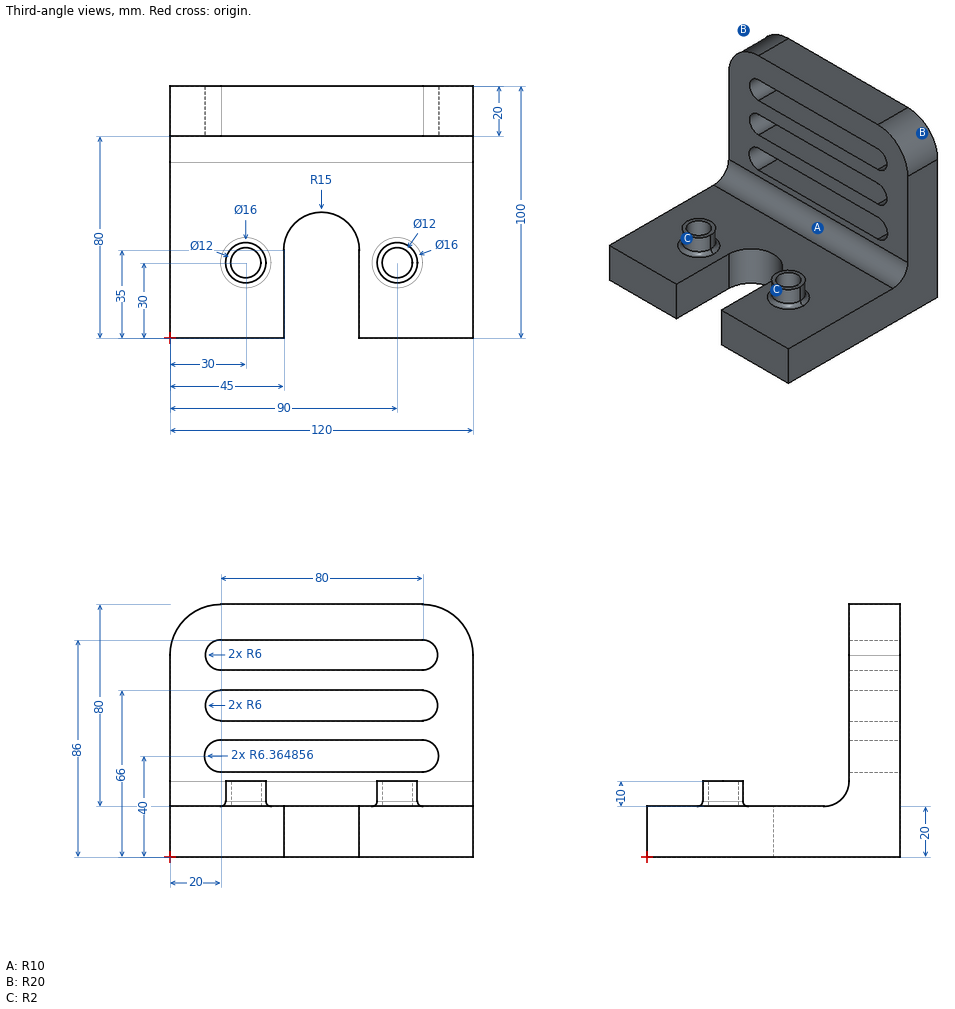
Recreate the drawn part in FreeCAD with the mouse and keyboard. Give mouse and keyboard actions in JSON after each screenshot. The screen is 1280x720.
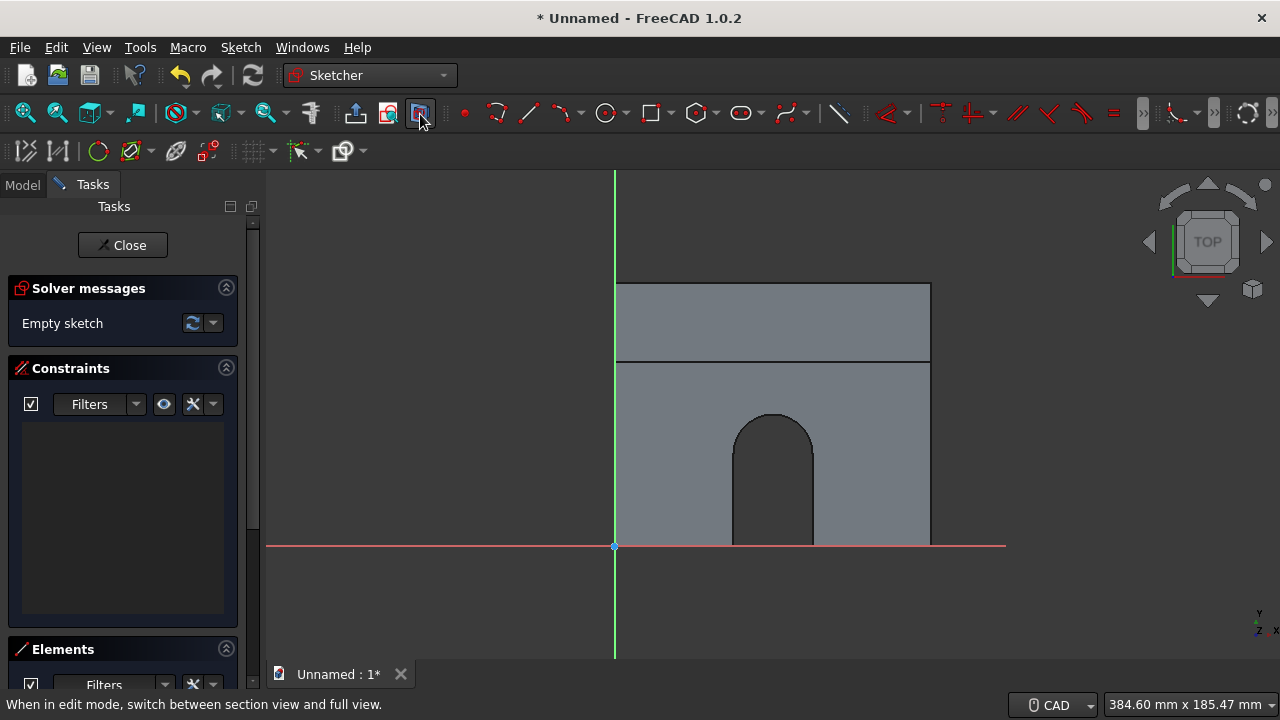
{"action": "scroll", "coordinate": [648, 531], "scroll_direction": "up", "scroll_amount": 6}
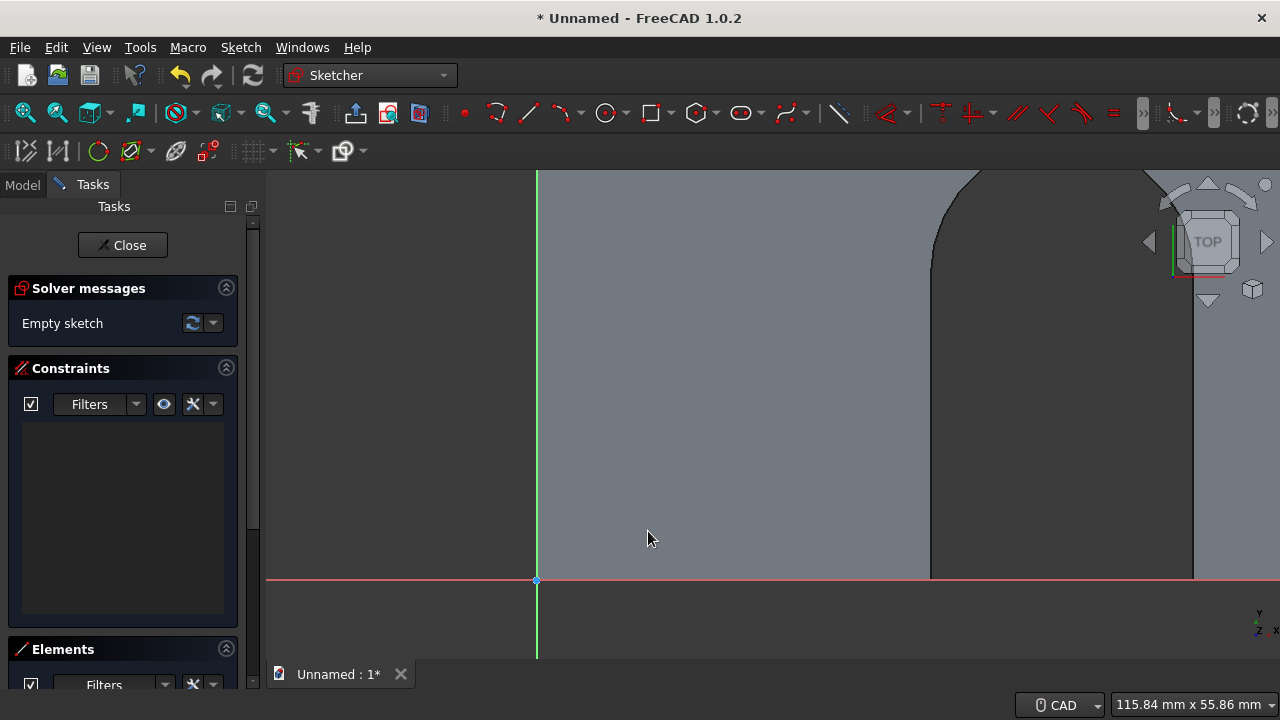
{"action": "left_click", "coordinate": [606, 114]}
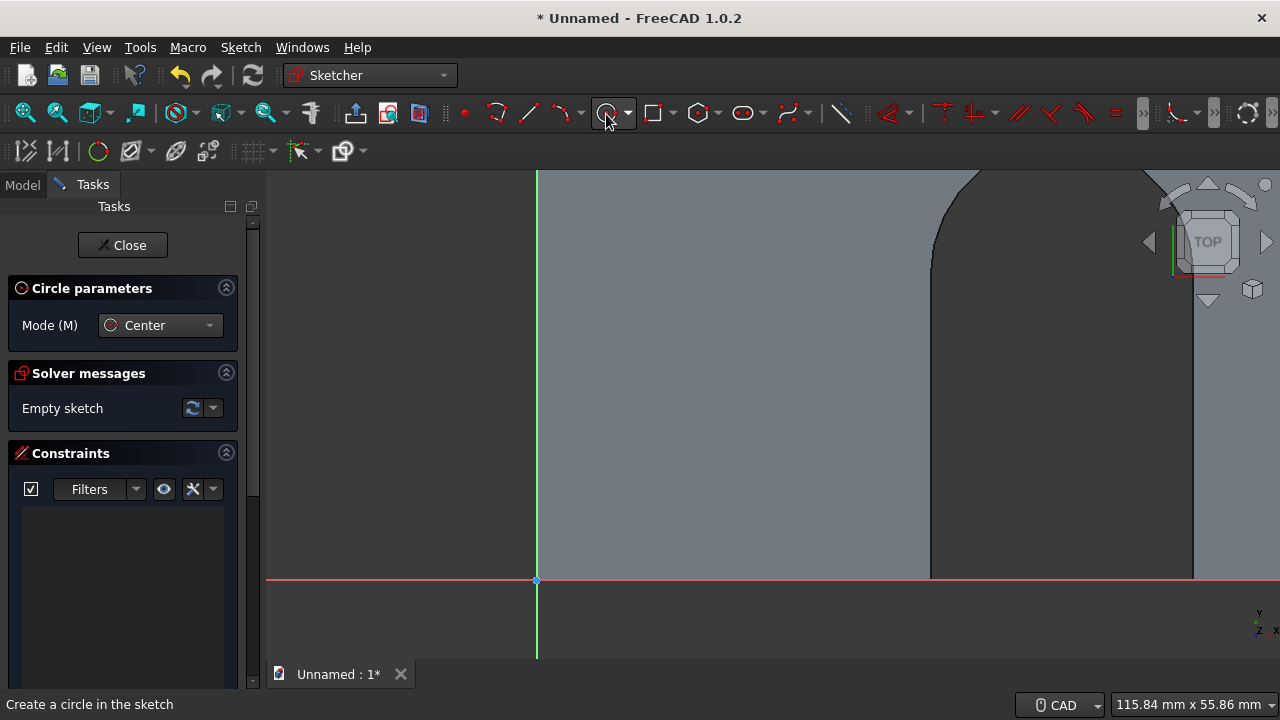
{"action": "left_click", "coordinate": [800, 318]}
{"action": "mouse_move", "coordinate": [849, 268]}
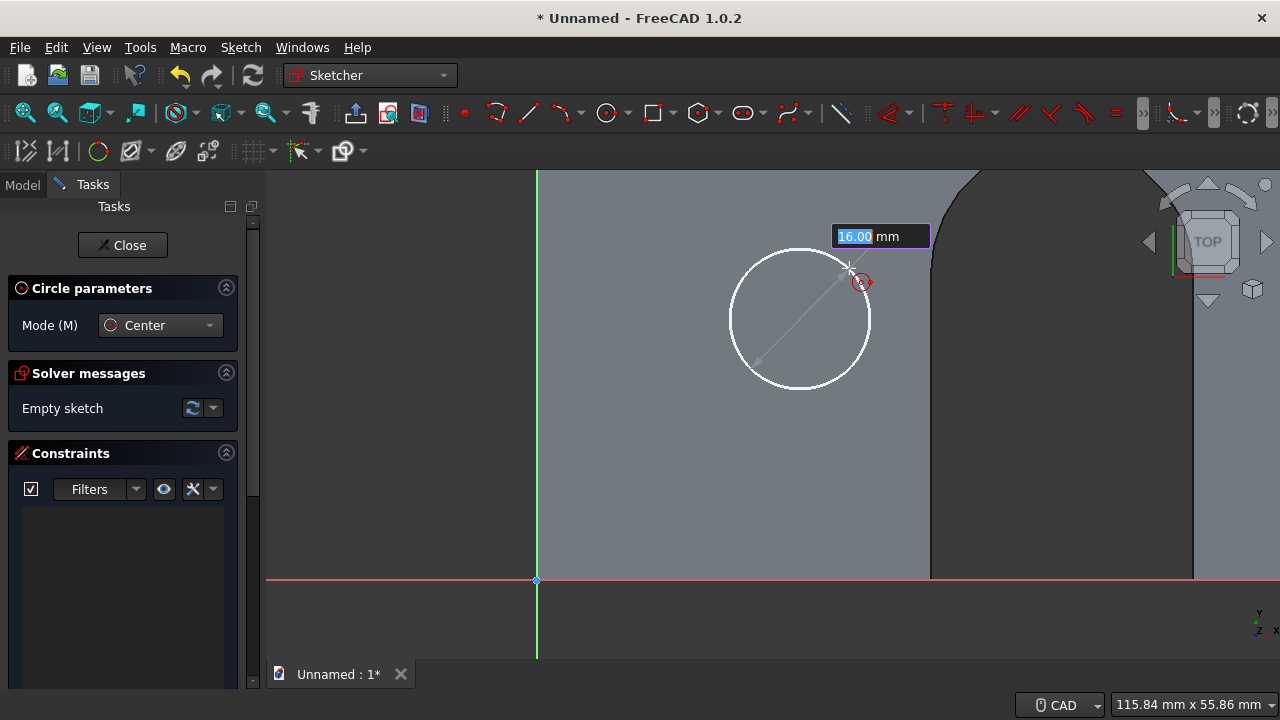
{"action": "type", "text": "16"}
{"action": "key", "text": "Return"}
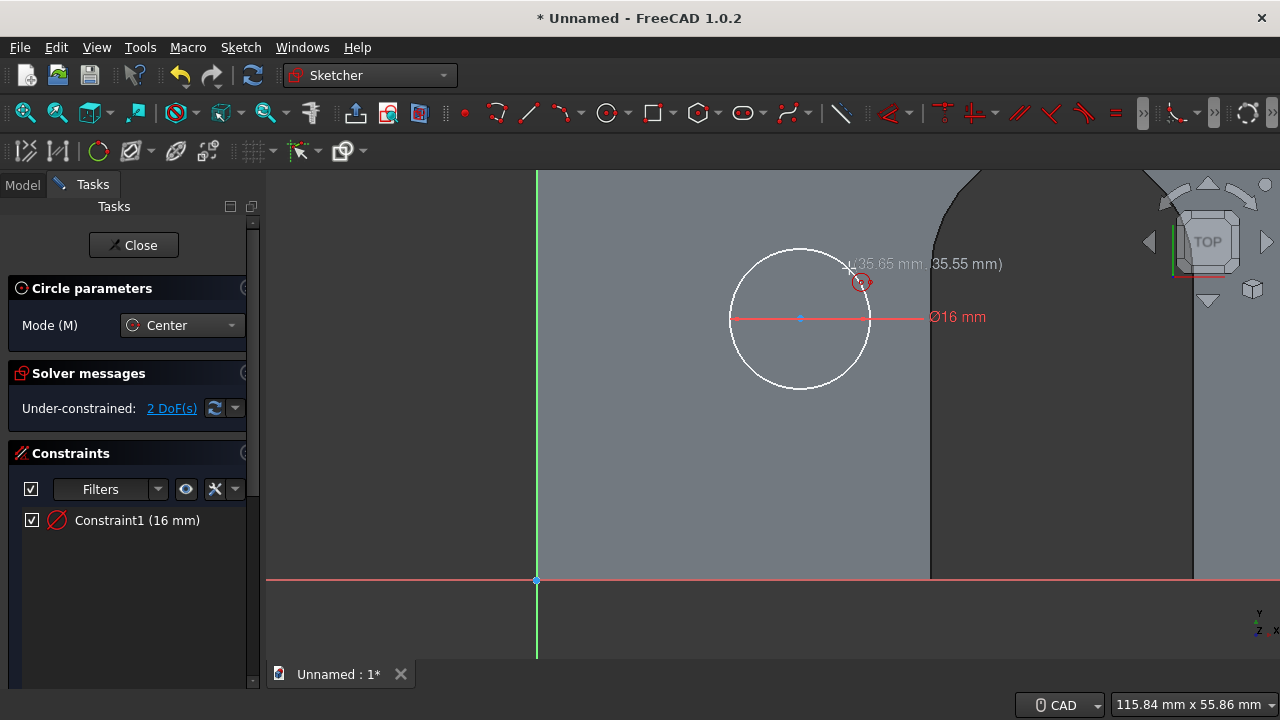
{"action": "left_click", "coordinate": [800, 319]}
{"action": "mouse_move", "coordinate": [837, 280]}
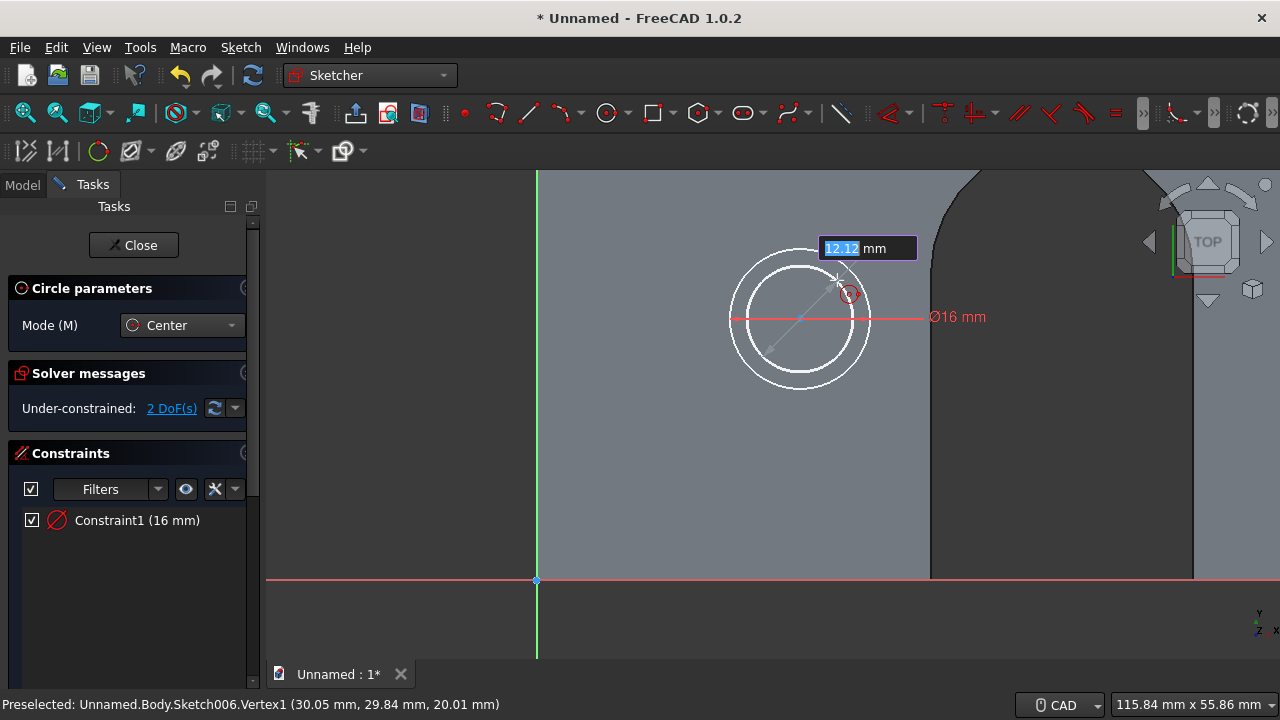
{"action": "type", "text": "12"}
{"action": "key", "text": "Return"}
{"action": "key", "text": "Escape"}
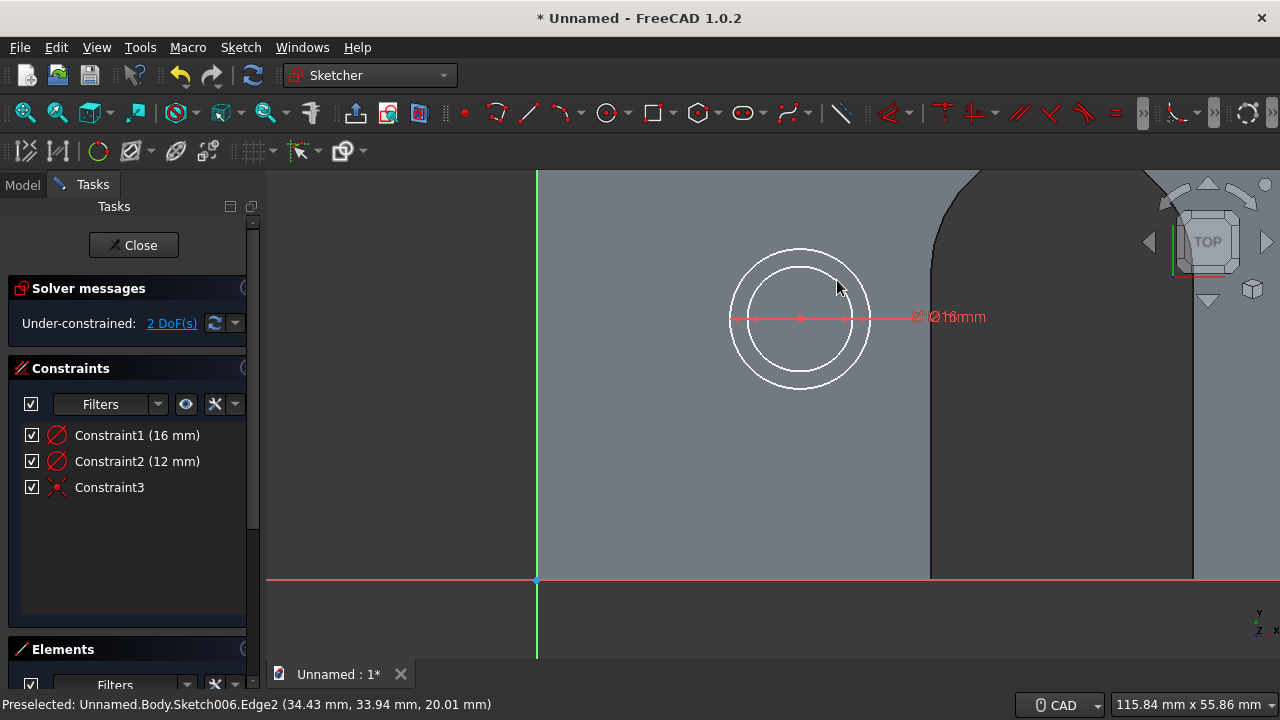
{"action": "left_click", "coordinate": [888, 114]}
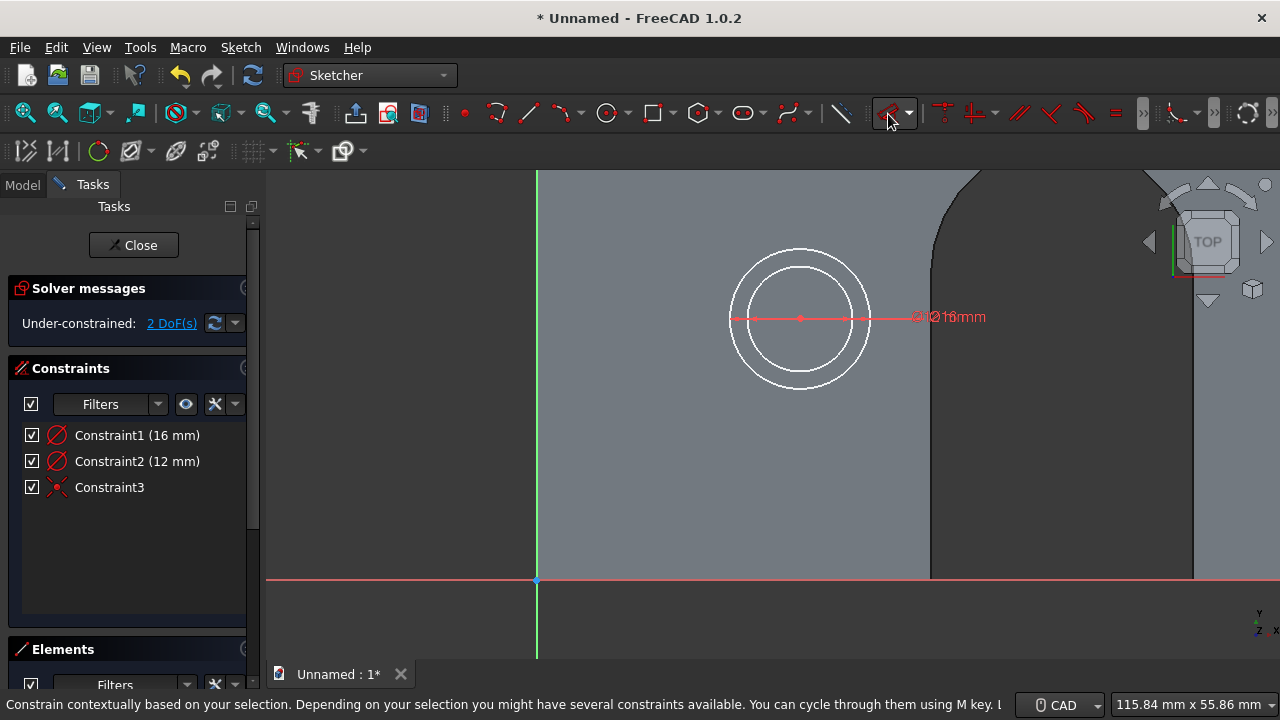
{"action": "left_click", "coordinate": [800, 319]}
{"action": "left_click", "coordinate": [668, 614]}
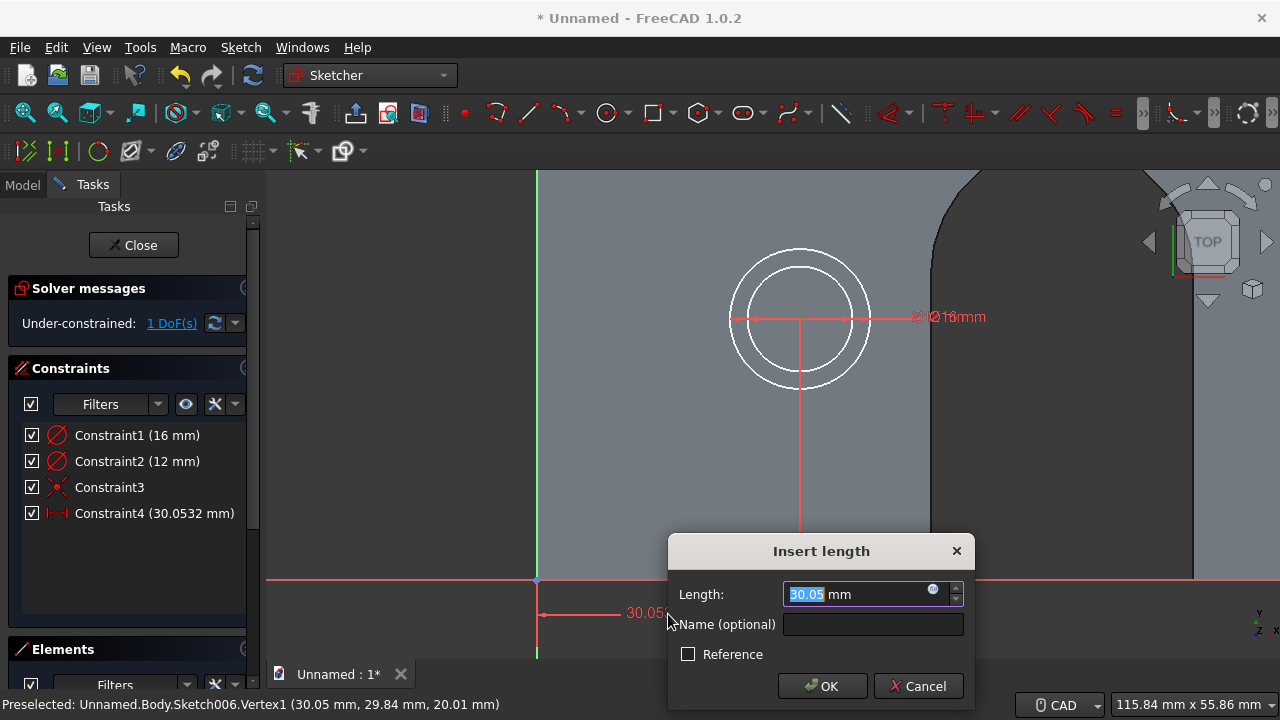
{"action": "type", "text": "30"}
{"action": "key", "text": "Return"}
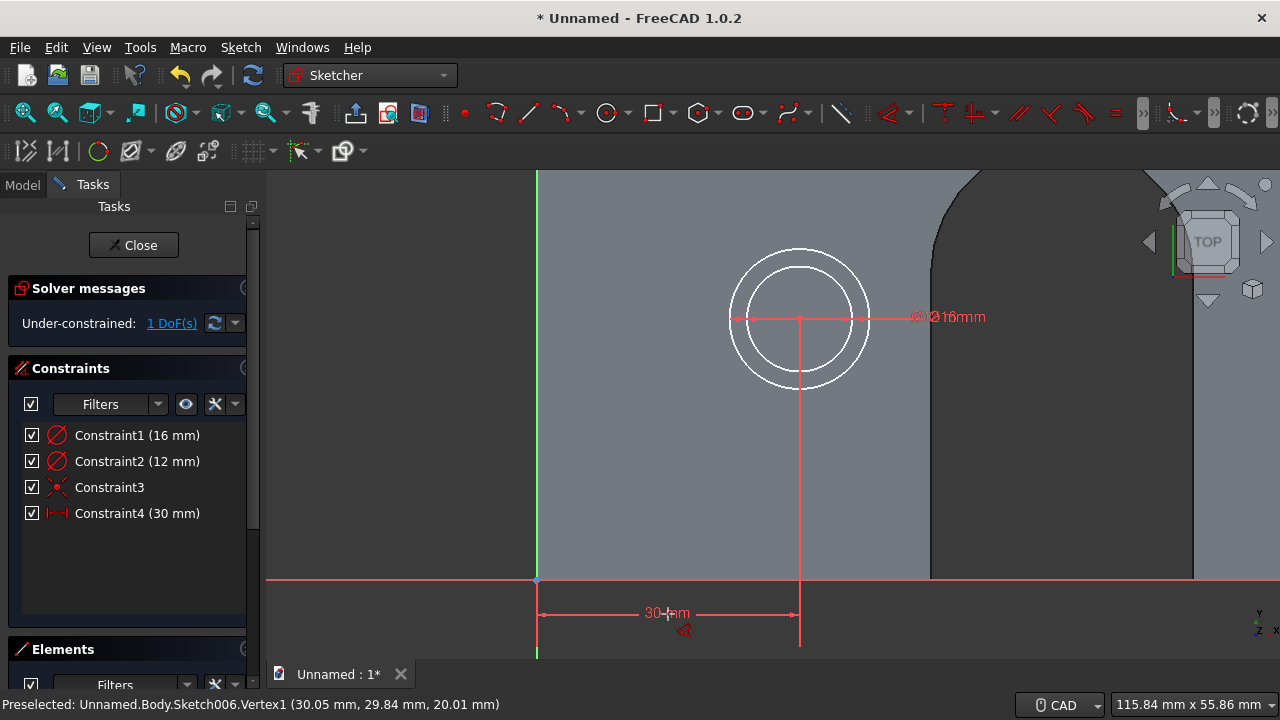
{"action": "left_click", "coordinate": [800, 319]}
{"action": "left_click", "coordinate": [503, 450]}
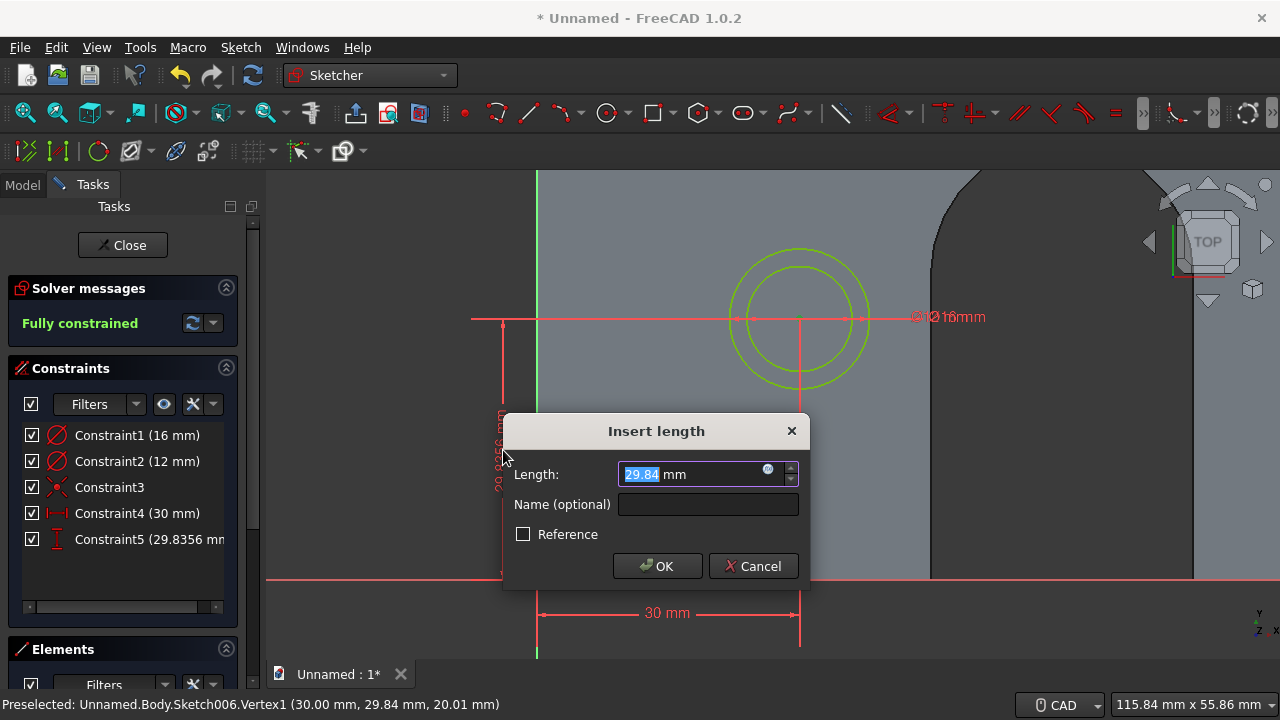
{"action": "type", "text": "30"}
{"action": "key", "text": "Return"}
{"action": "key", "text": "Escape"}